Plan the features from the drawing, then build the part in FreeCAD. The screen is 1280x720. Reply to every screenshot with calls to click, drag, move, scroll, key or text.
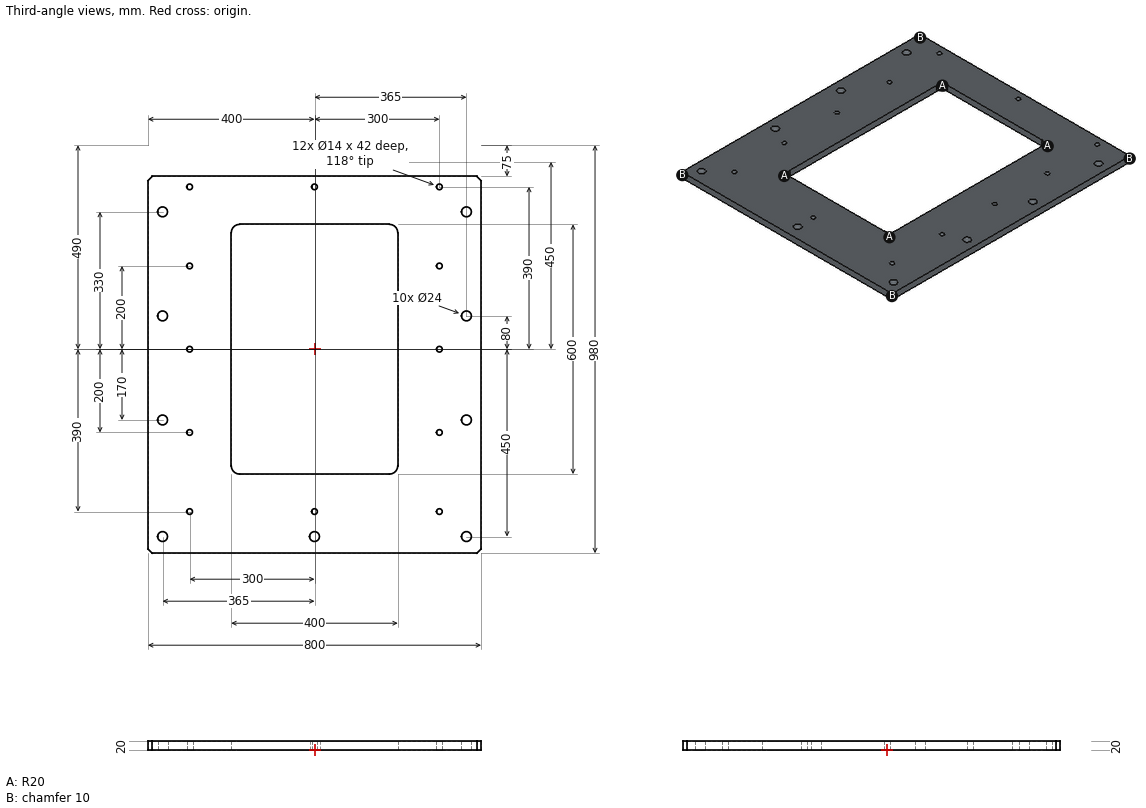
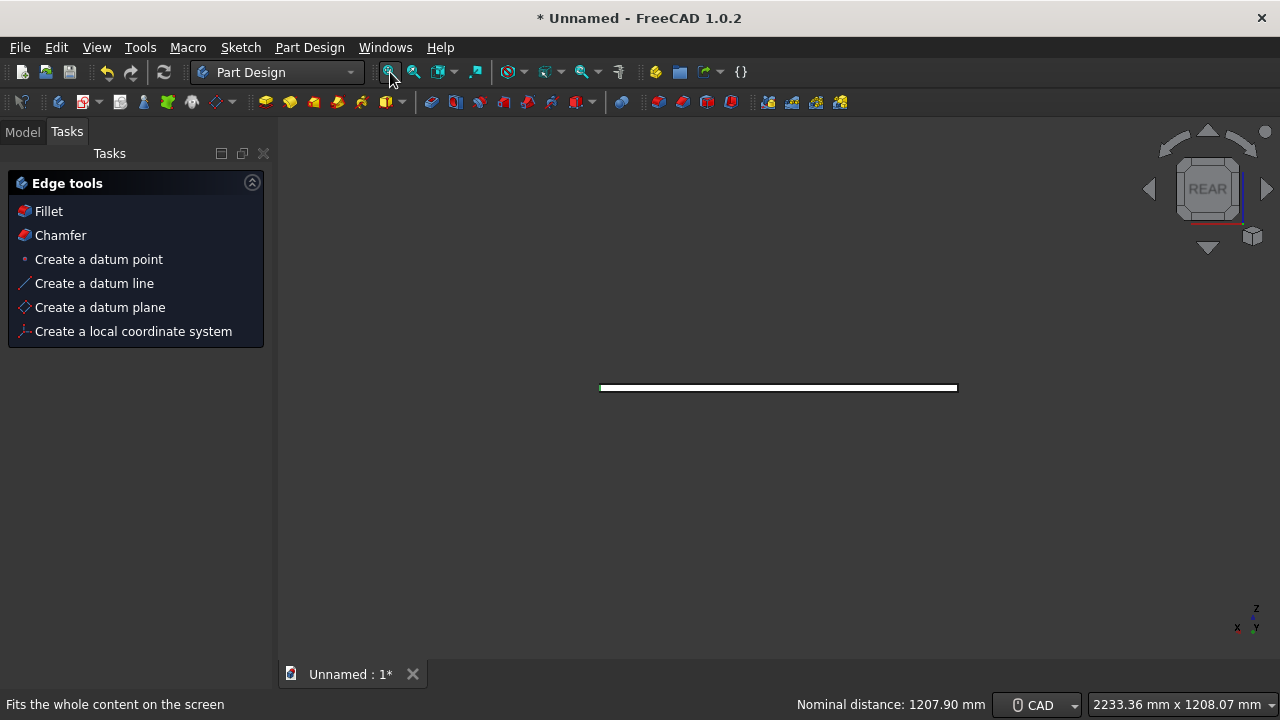
click(390, 72)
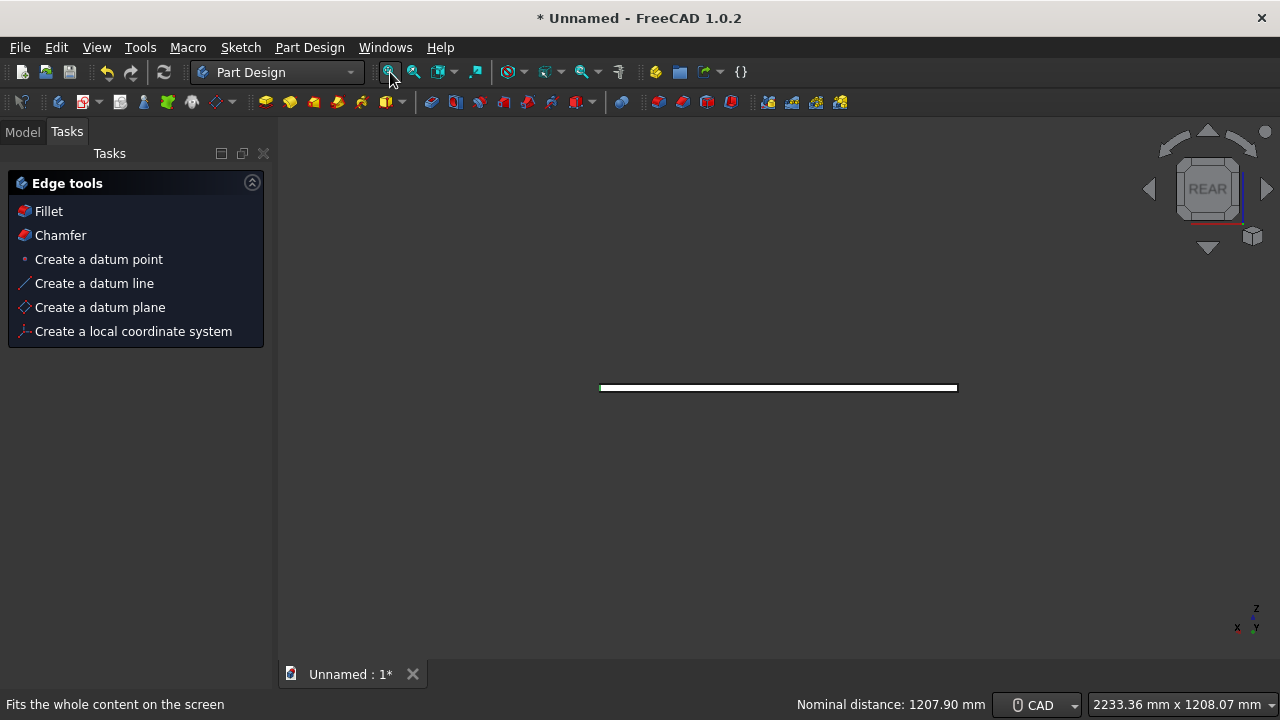
scroll(958, 387, up, 8)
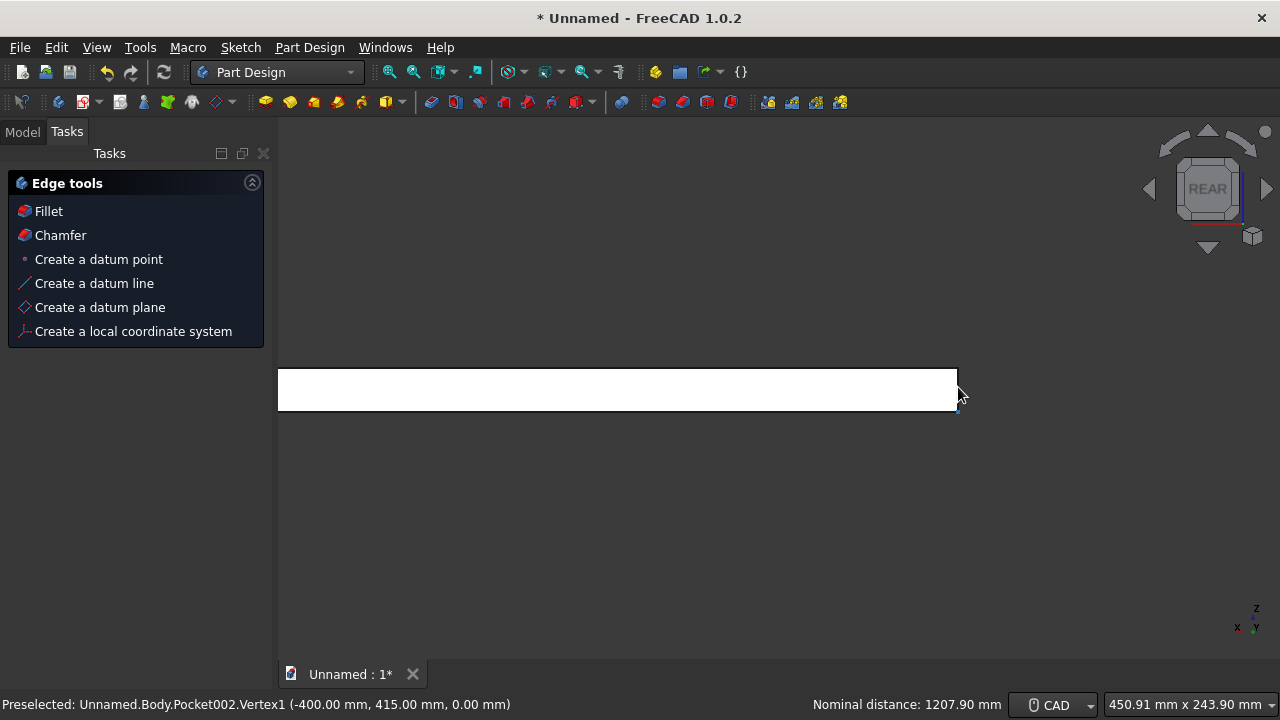
click(958, 389, ctrl)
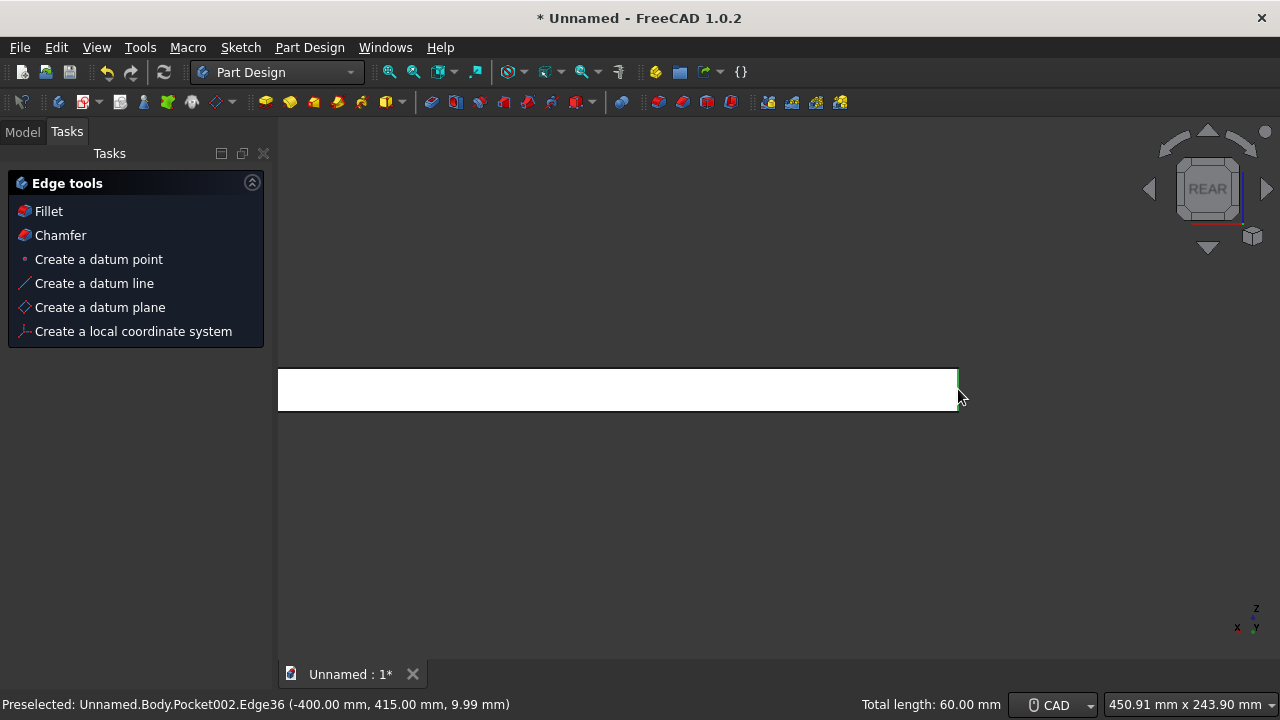
click(390, 72)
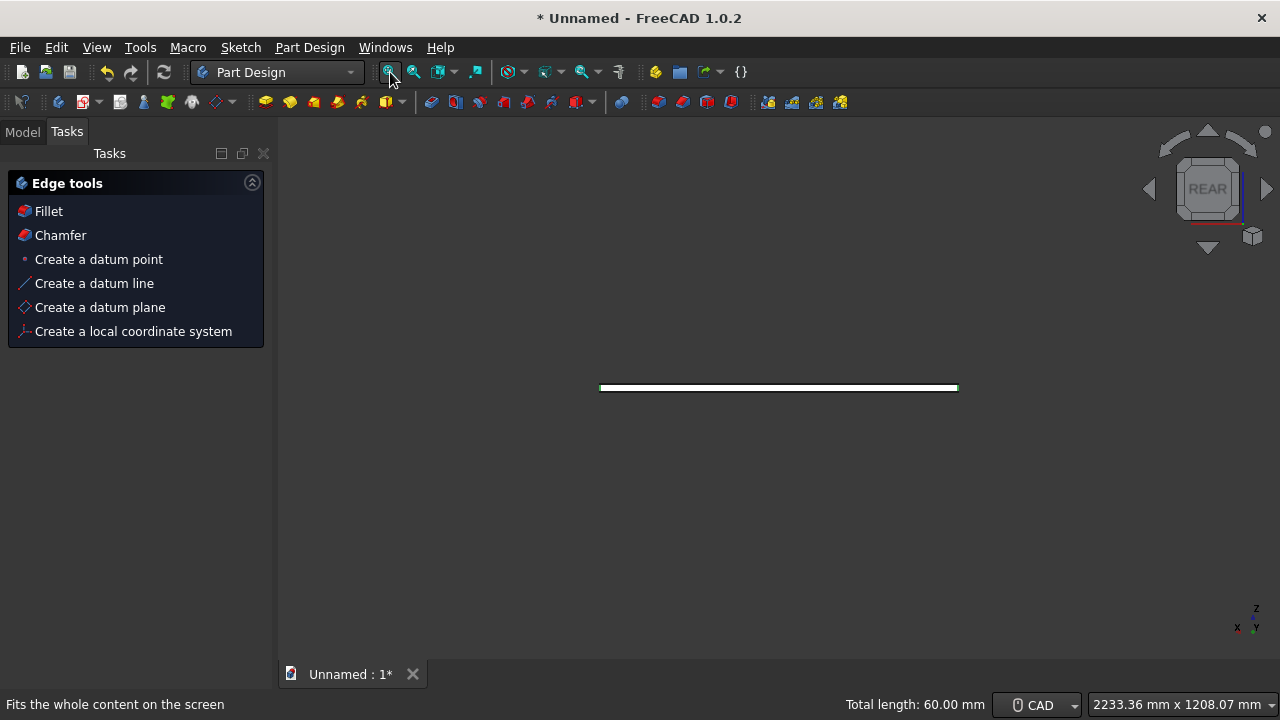
key(6)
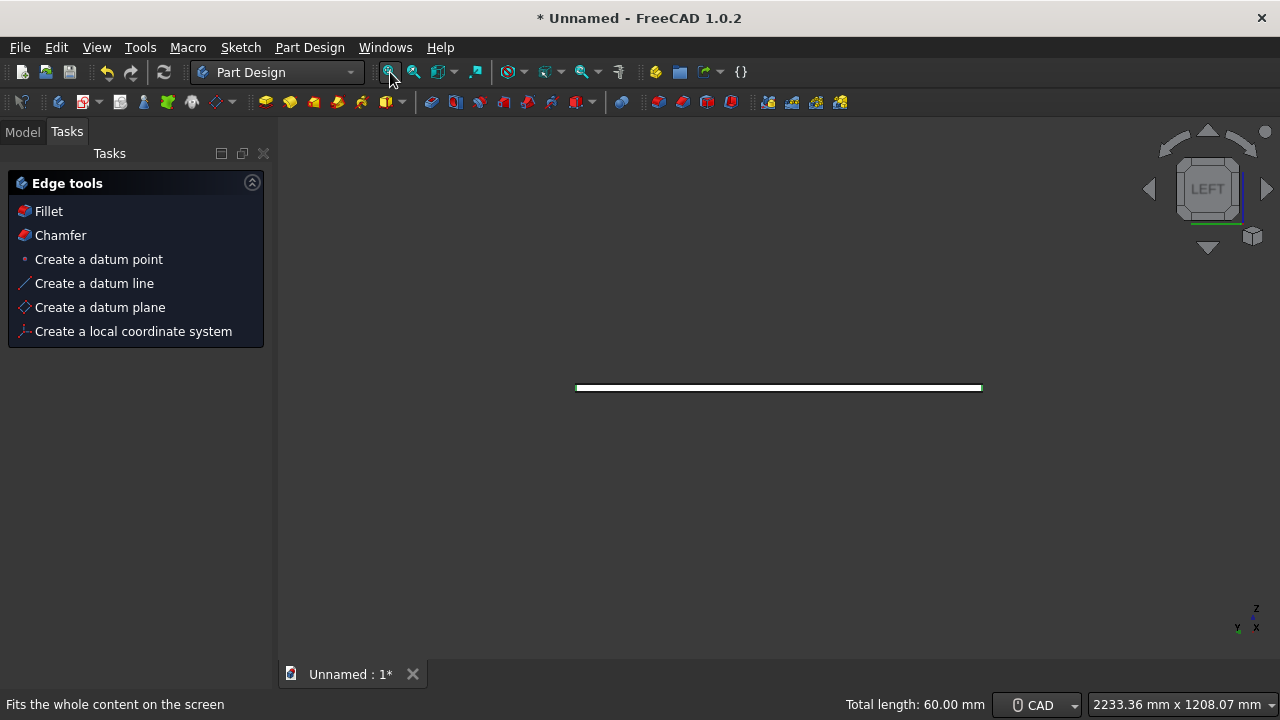
click(390, 72)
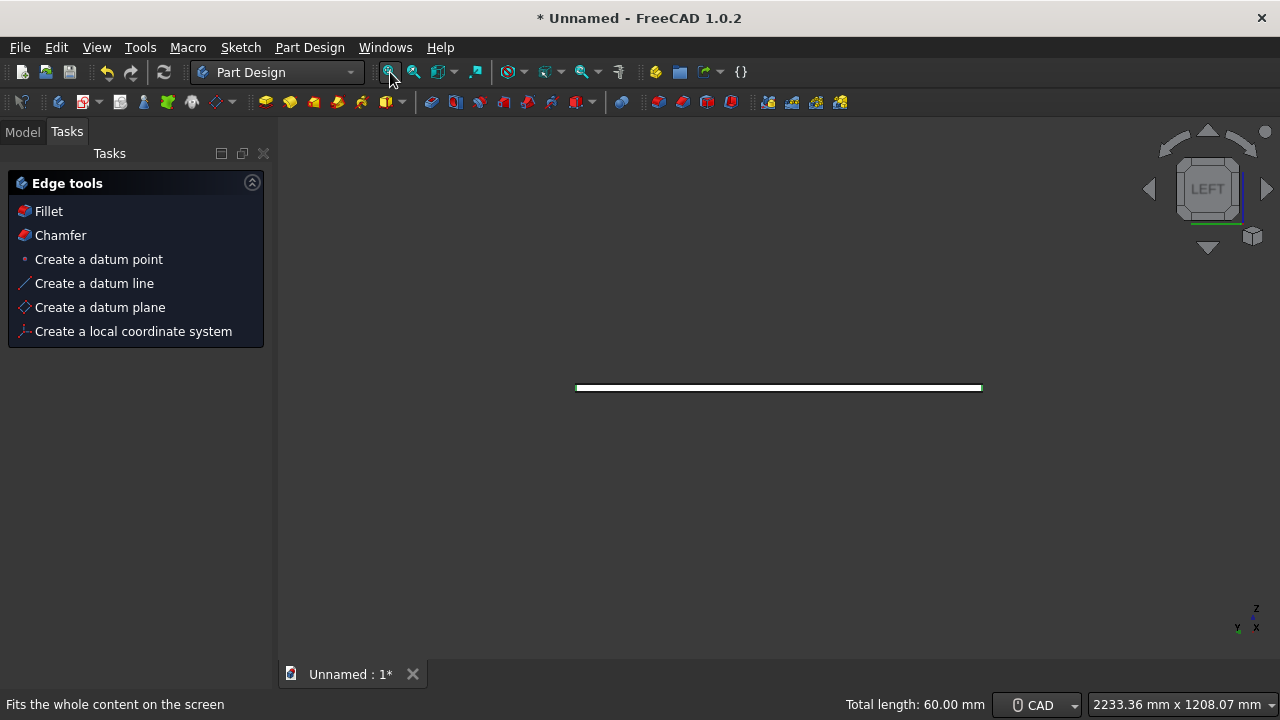
scroll(982, 387, up, 8)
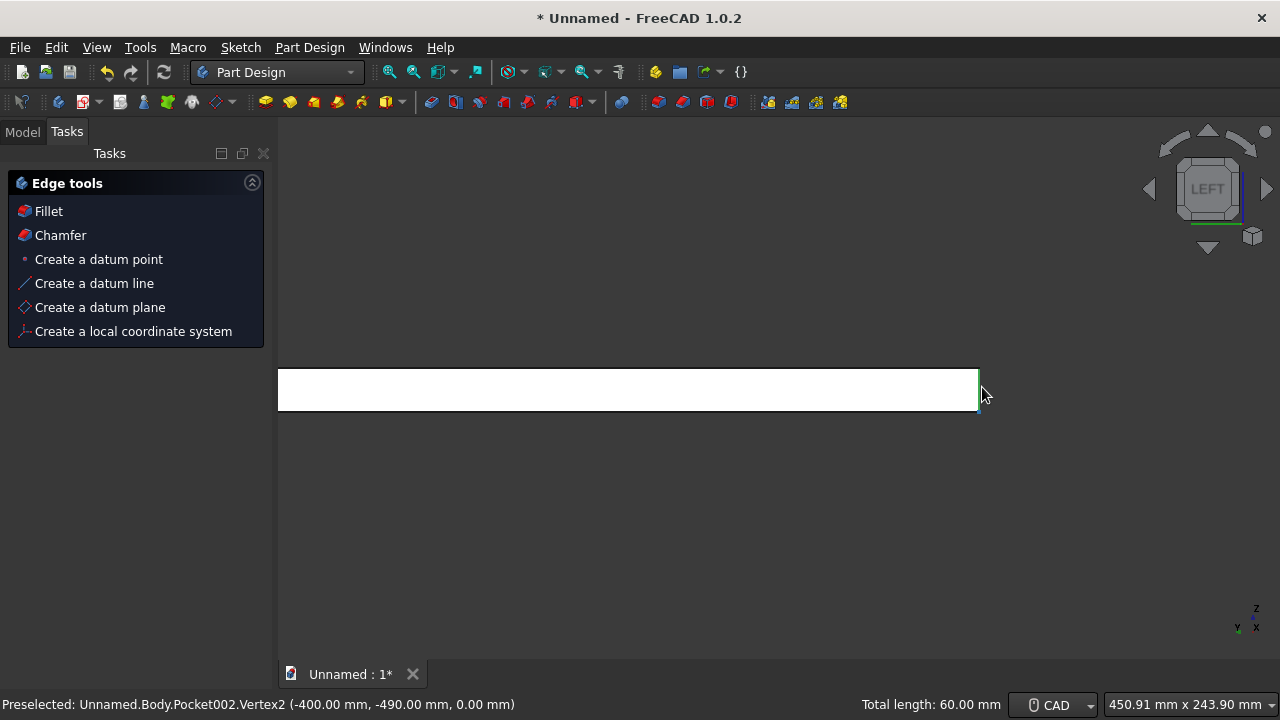
click(390, 72)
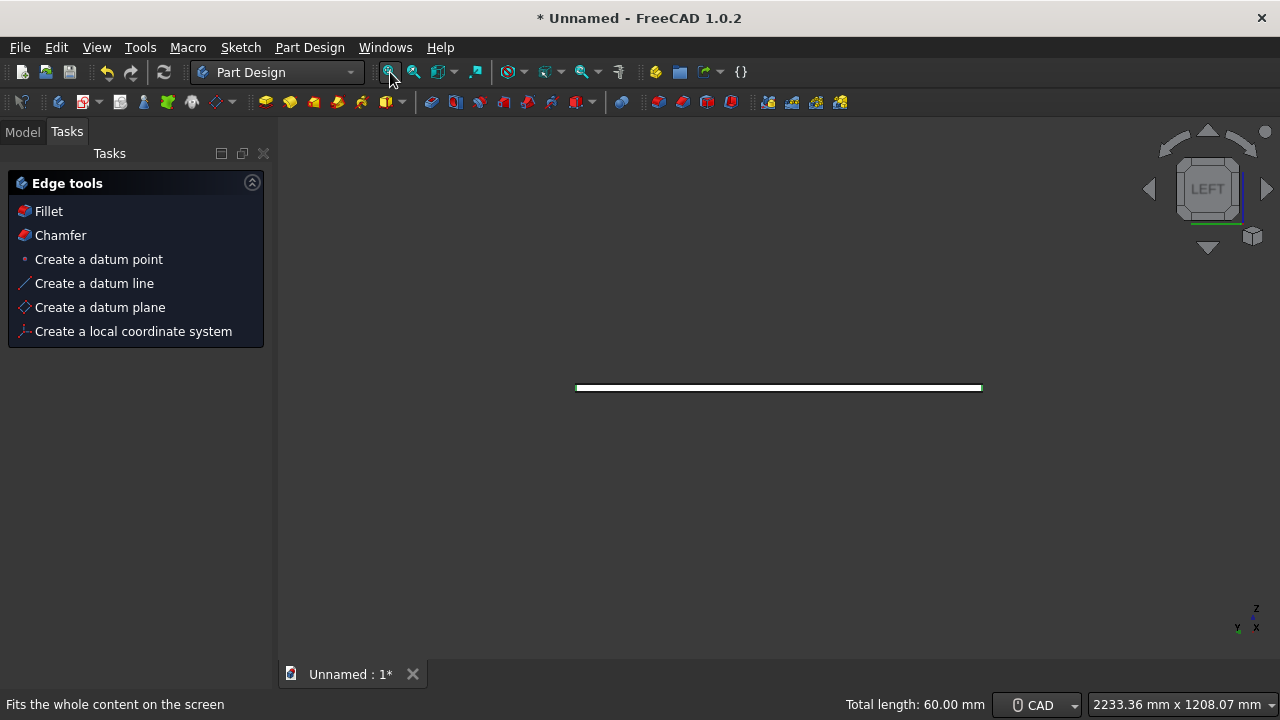
key(v)
key(3)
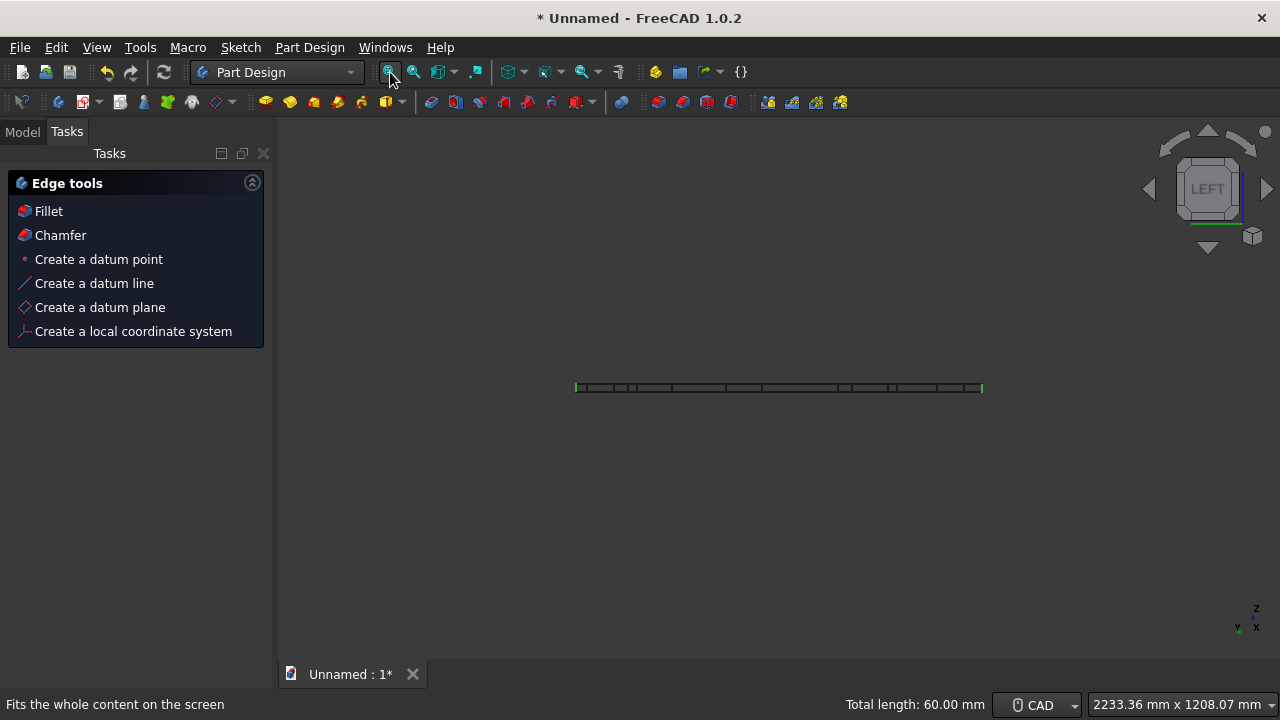
key(0)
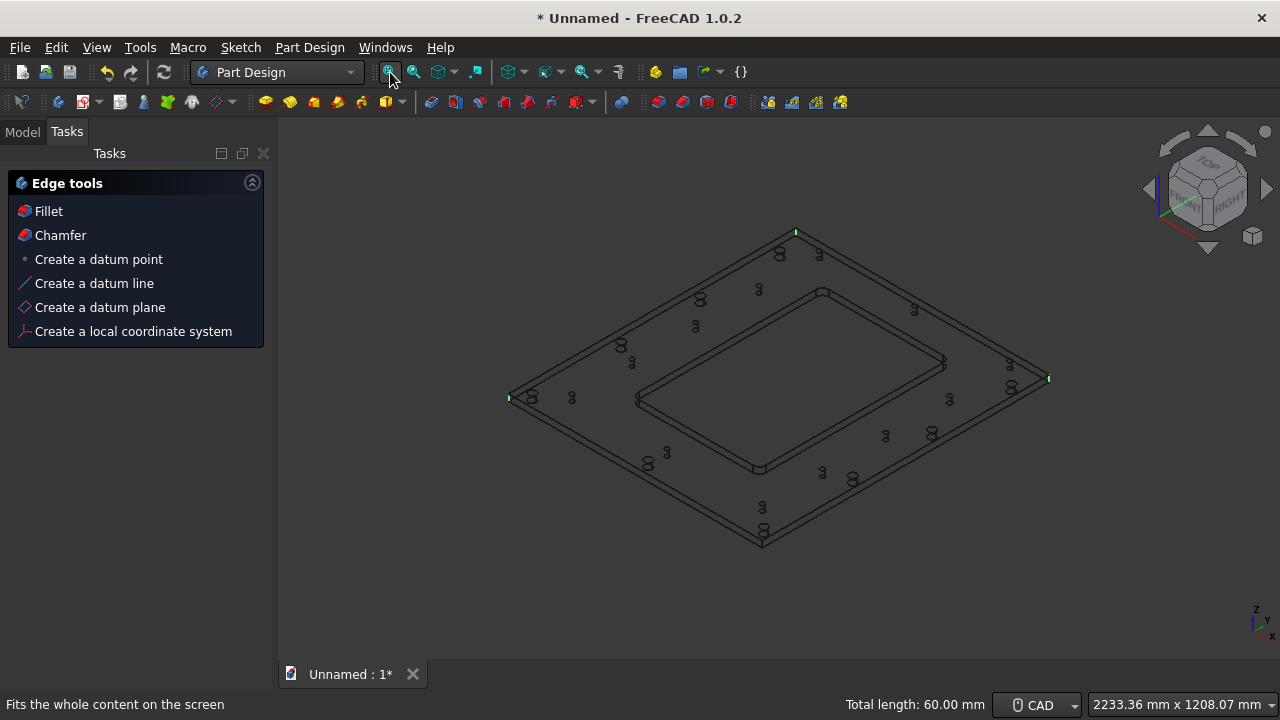
scroll(762, 543, up, 8)